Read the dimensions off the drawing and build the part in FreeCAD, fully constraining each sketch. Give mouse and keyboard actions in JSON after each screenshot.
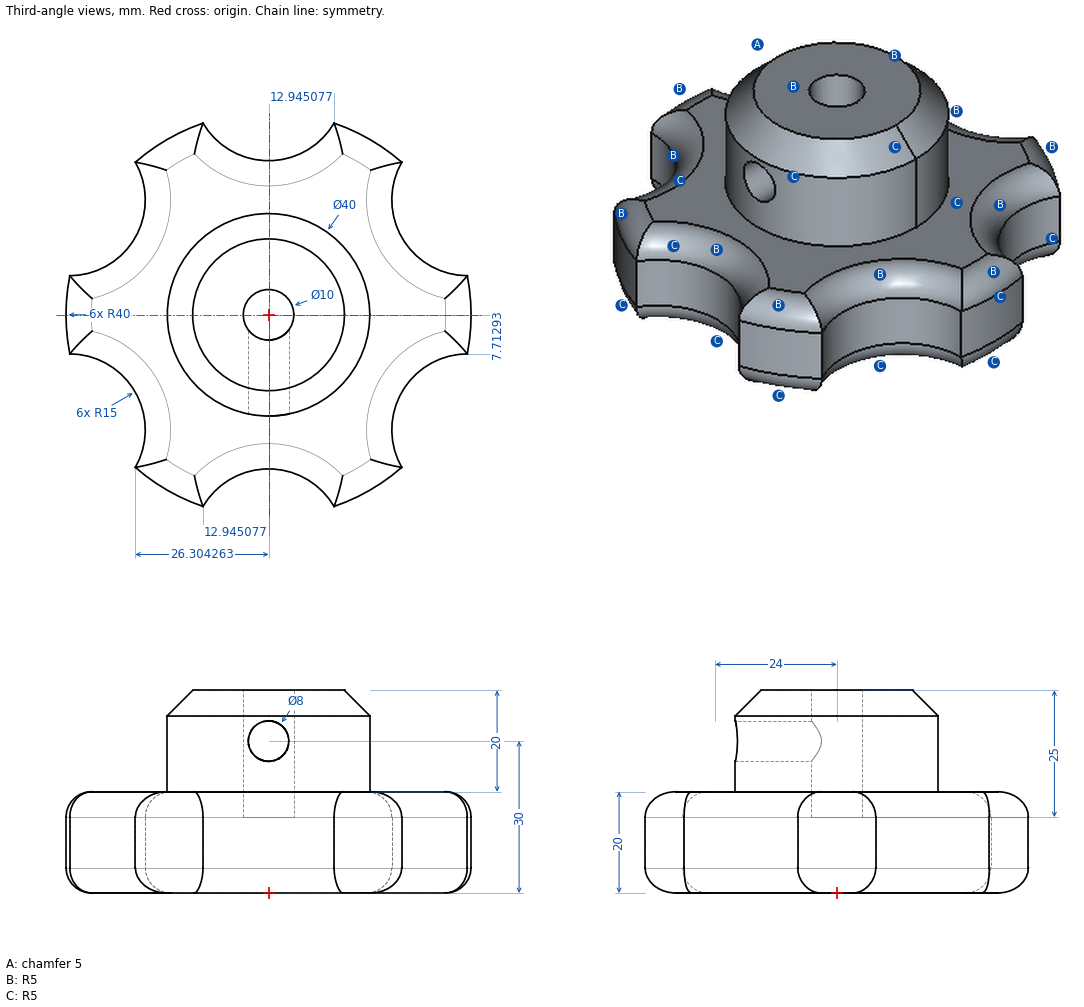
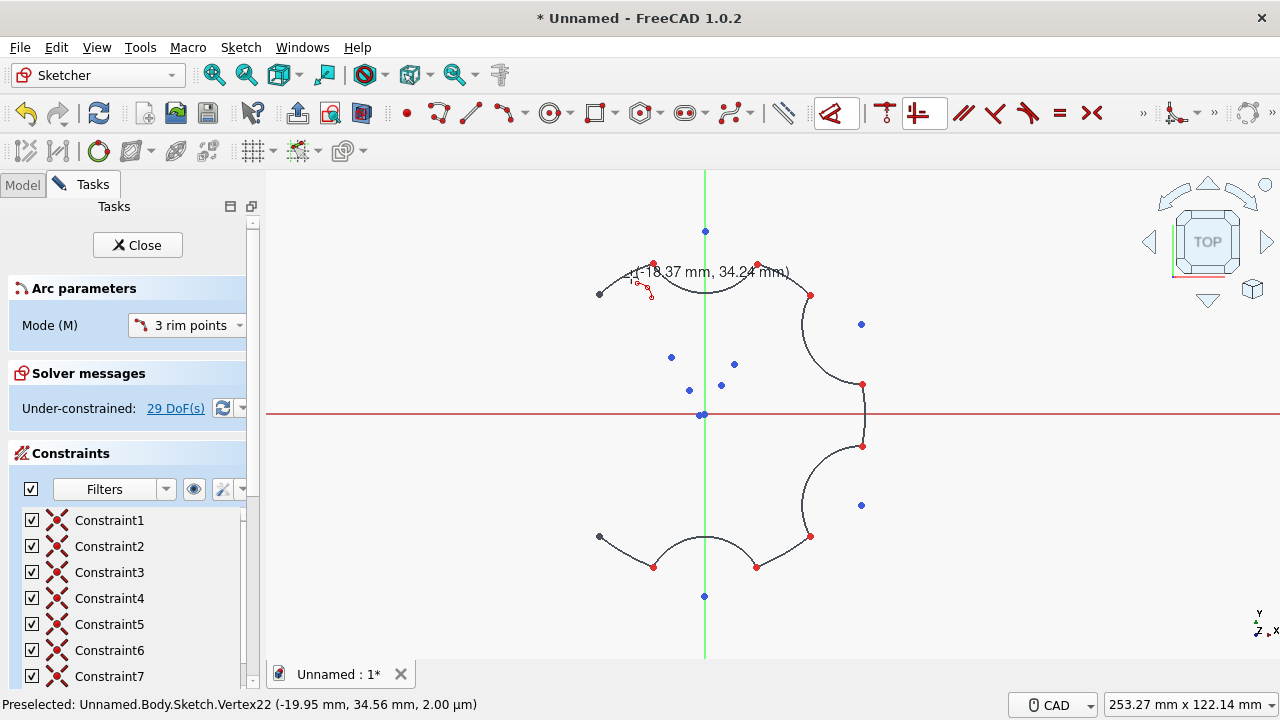
{"action": "left_click", "coordinate": [600, 294]}
{"action": "left_click", "coordinate": [548, 384]}
{"action": "left_click", "coordinate": [599, 354]}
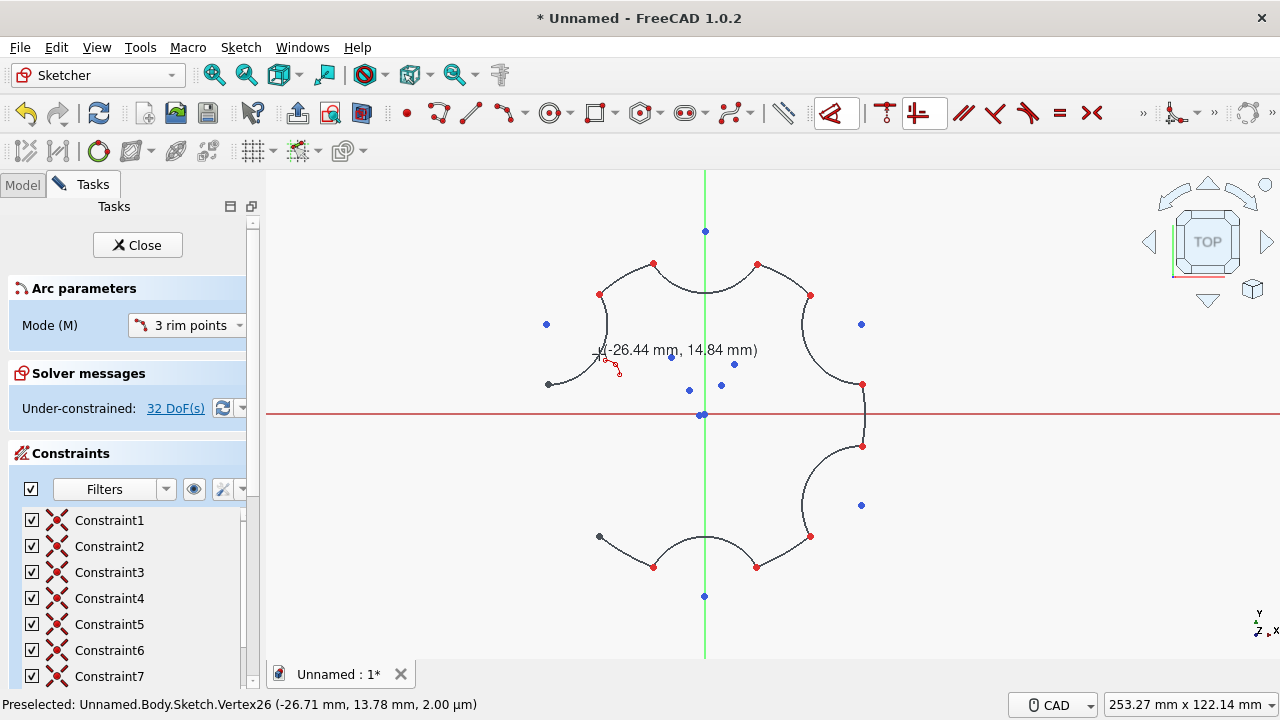
{"action": "left_click", "coordinate": [548, 385]}
{"action": "left_click", "coordinate": [548, 445]}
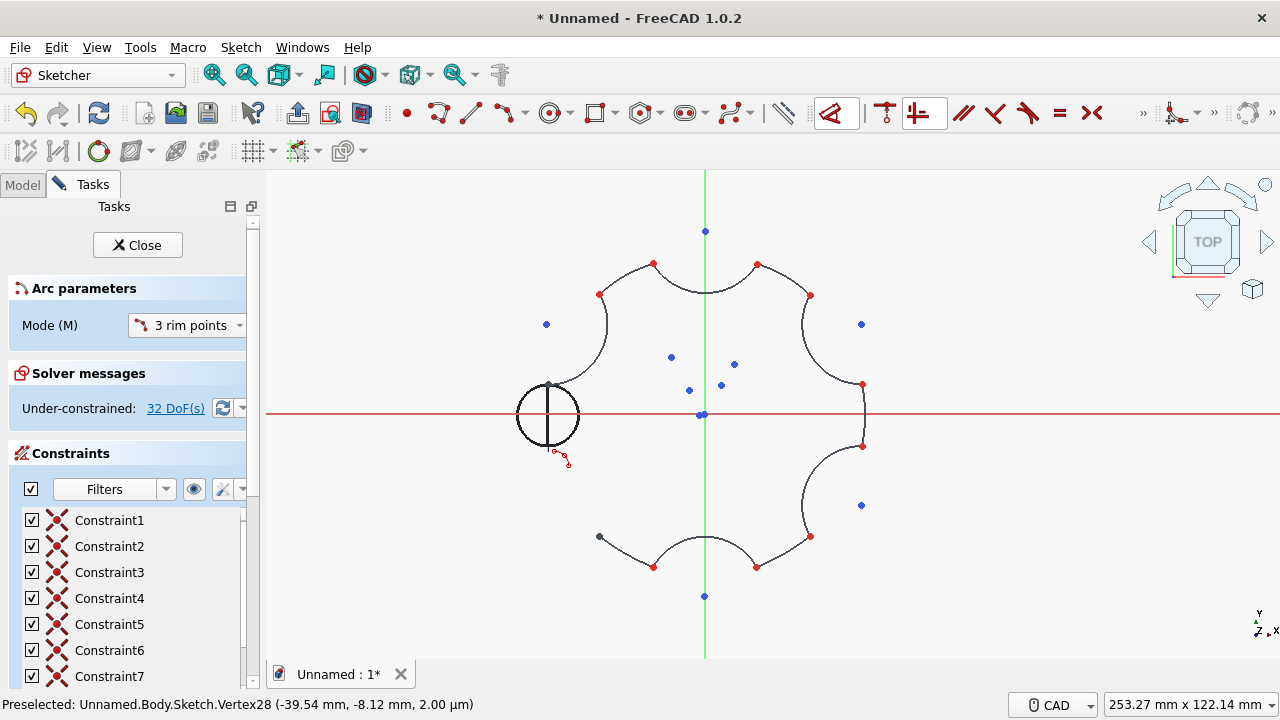
{"action": "scroll", "coordinate": [545, 408], "scroll_direction": "up", "scroll_amount": 9}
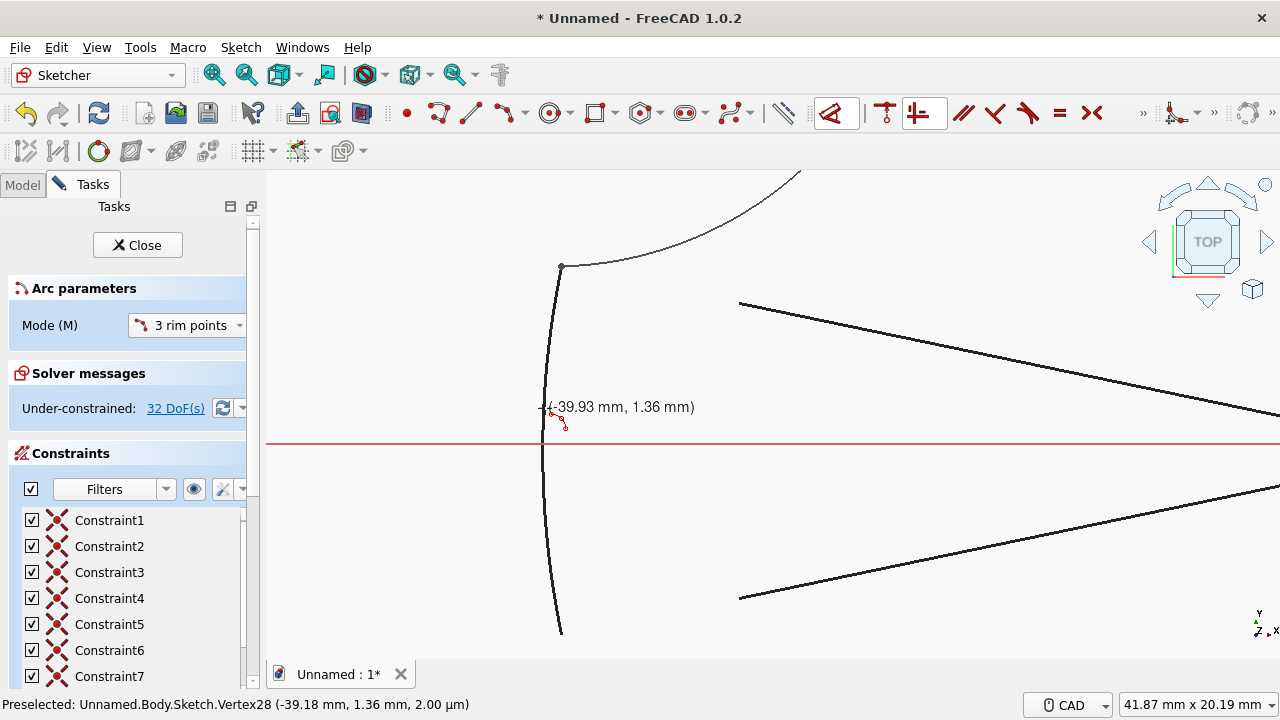
{"action": "left_click", "coordinate": [543, 407]}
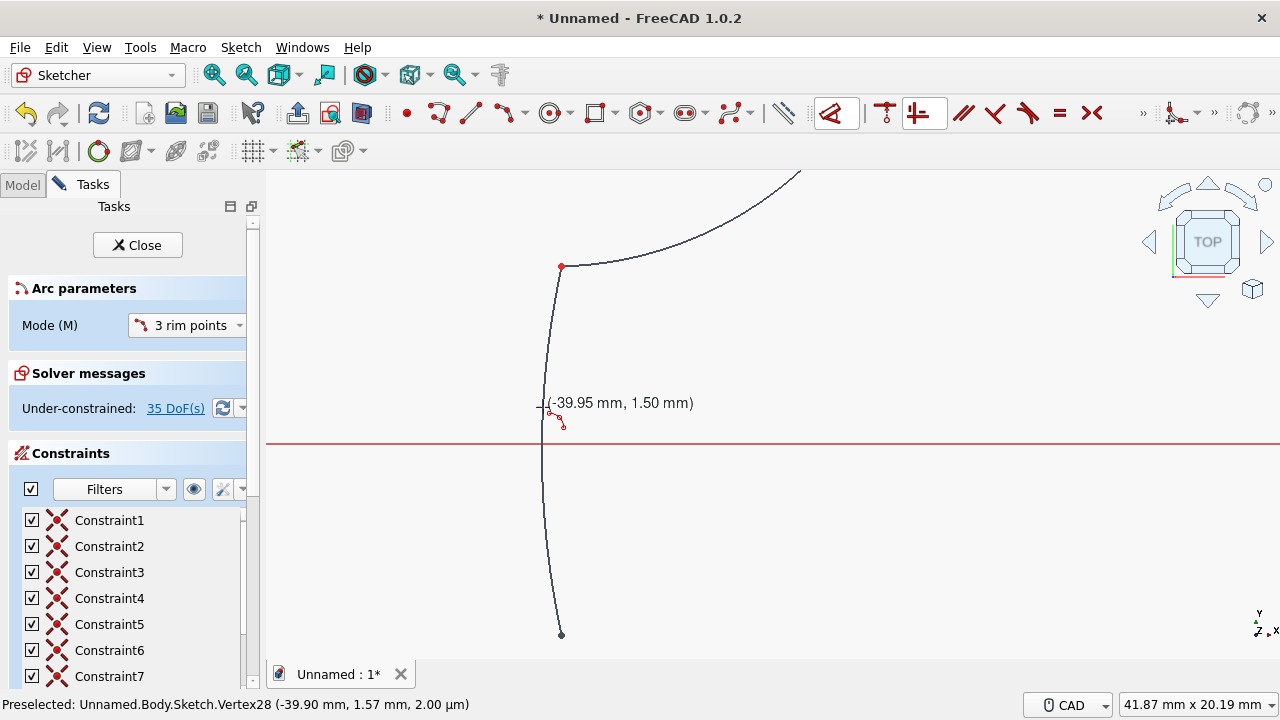
{"action": "scroll", "coordinate": [545, 409], "scroll_direction": "down", "scroll_amount": 9}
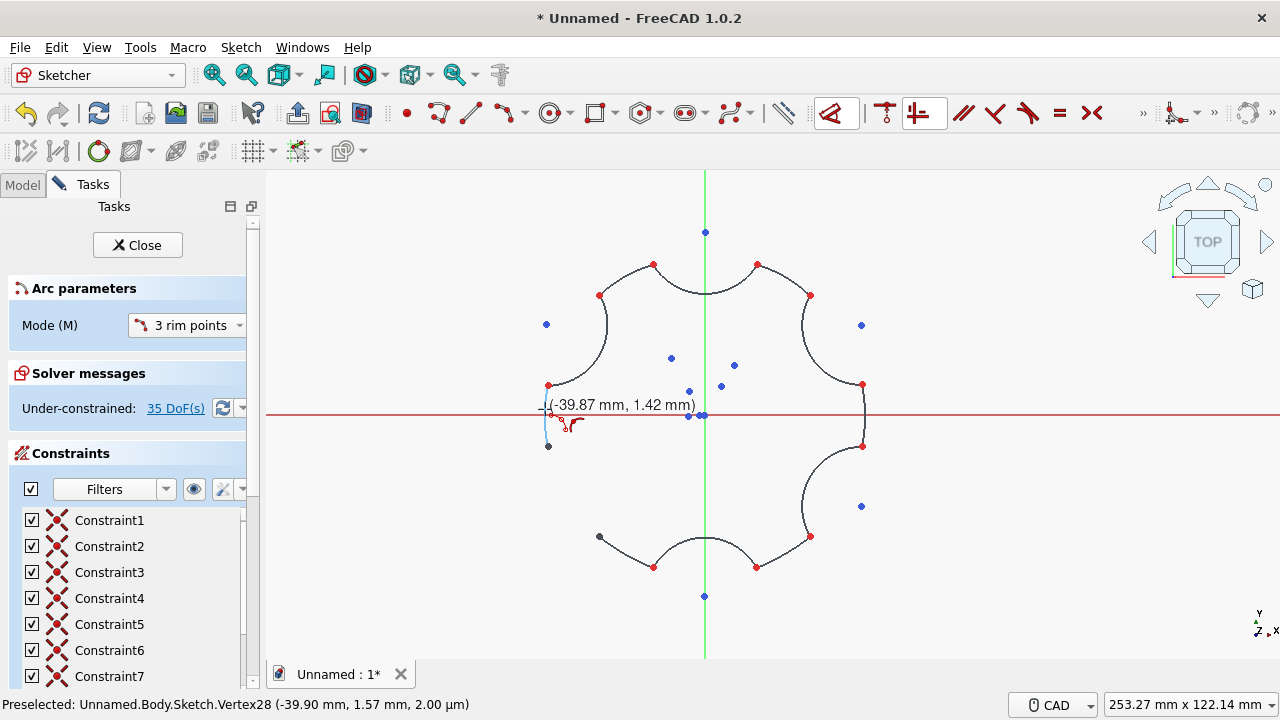
{"action": "left_click", "coordinate": [548, 447]}
{"action": "left_click", "coordinate": [599, 537]}
{"action": "left_click", "coordinate": [599, 476]}
{"action": "key", "text": "Escape"}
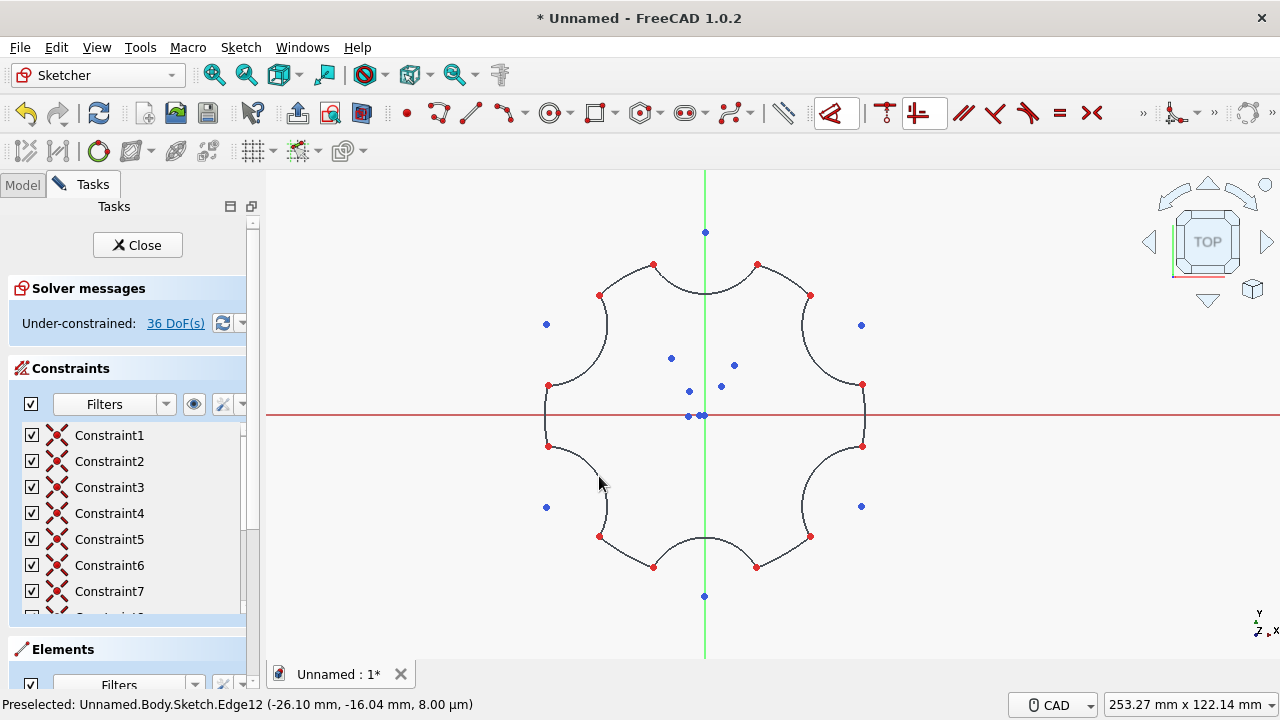
{"action": "left_click", "coordinate": [614, 548]}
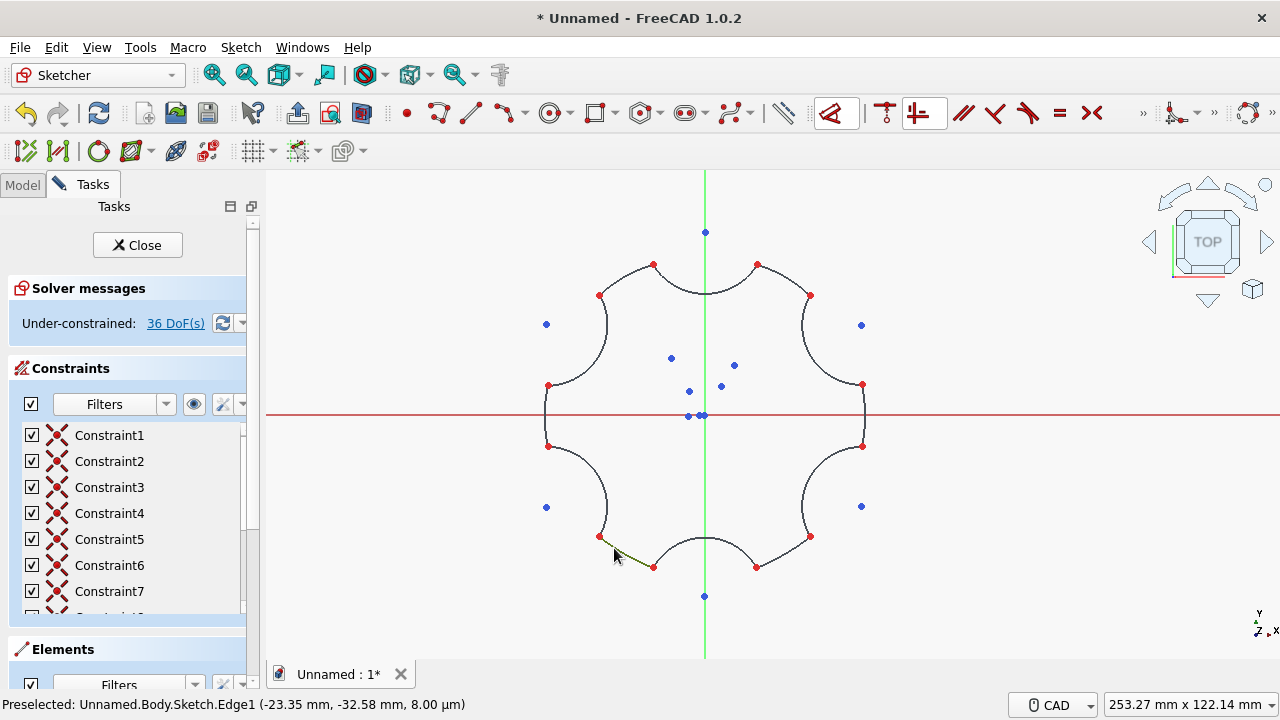
{"action": "left_click", "coordinate": [774, 560]}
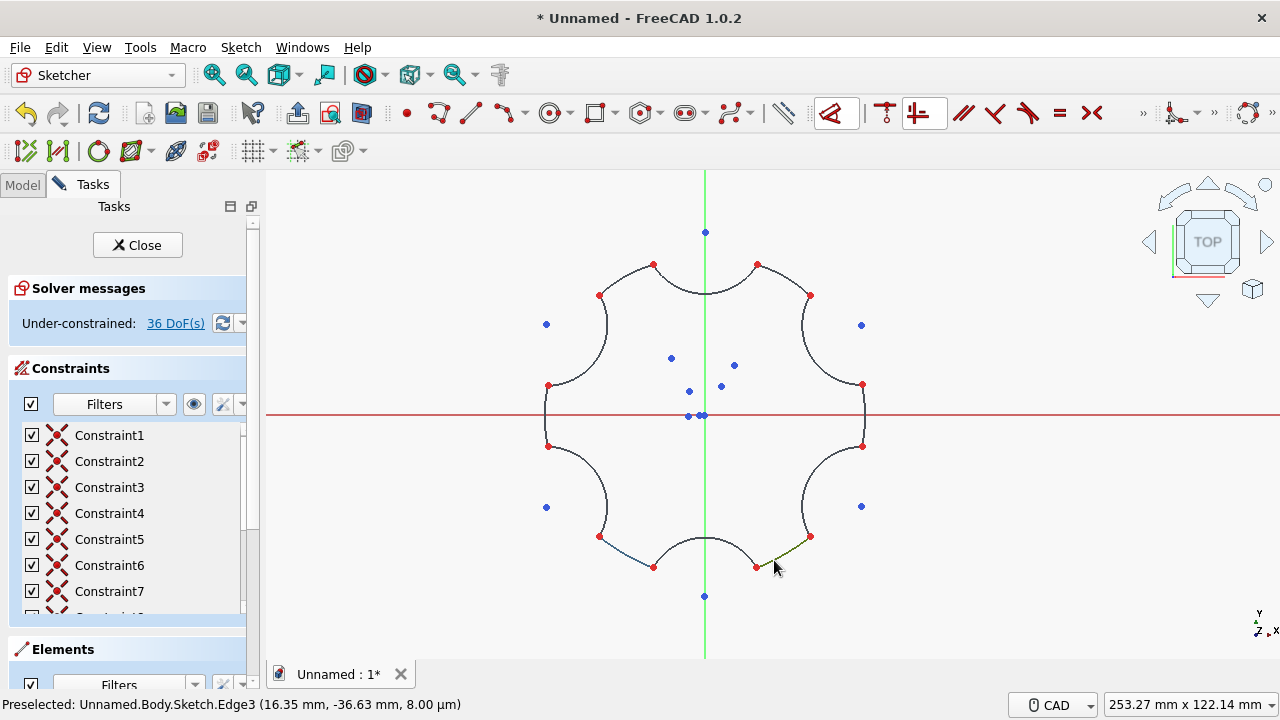
{"action": "left_click", "coordinate": [886, 114]}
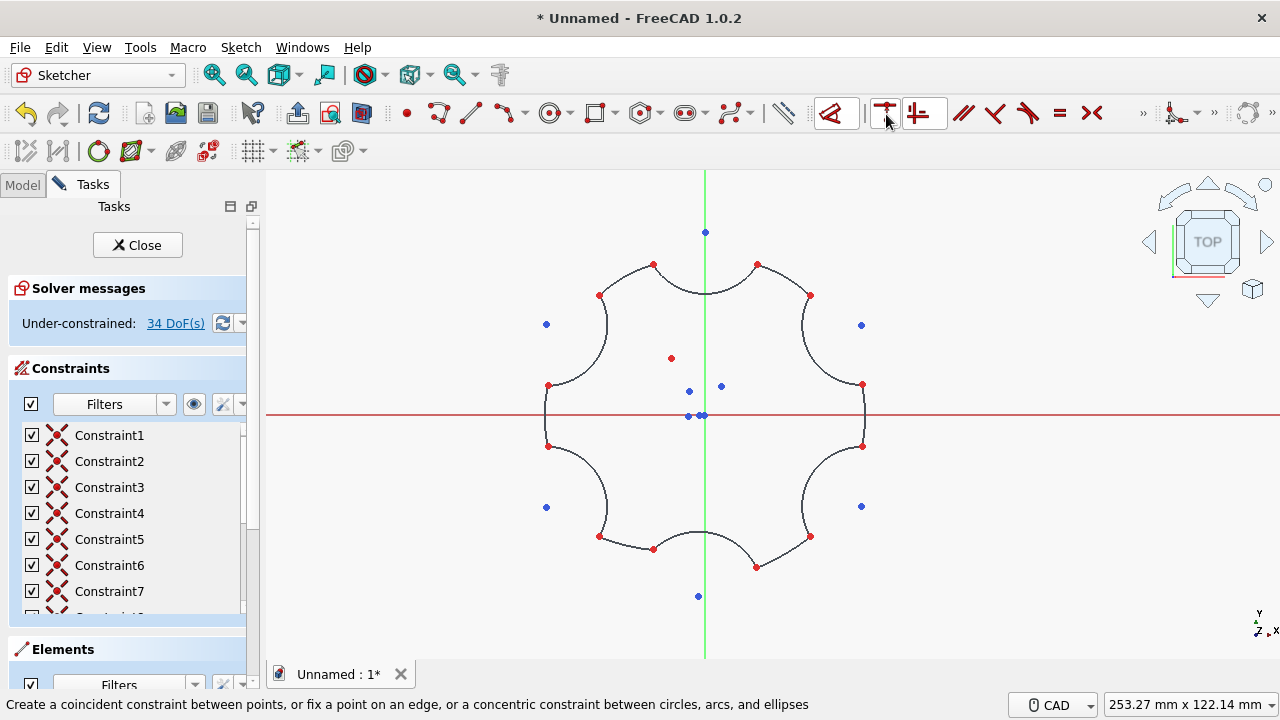
{"action": "left_click", "coordinate": [615, 542]}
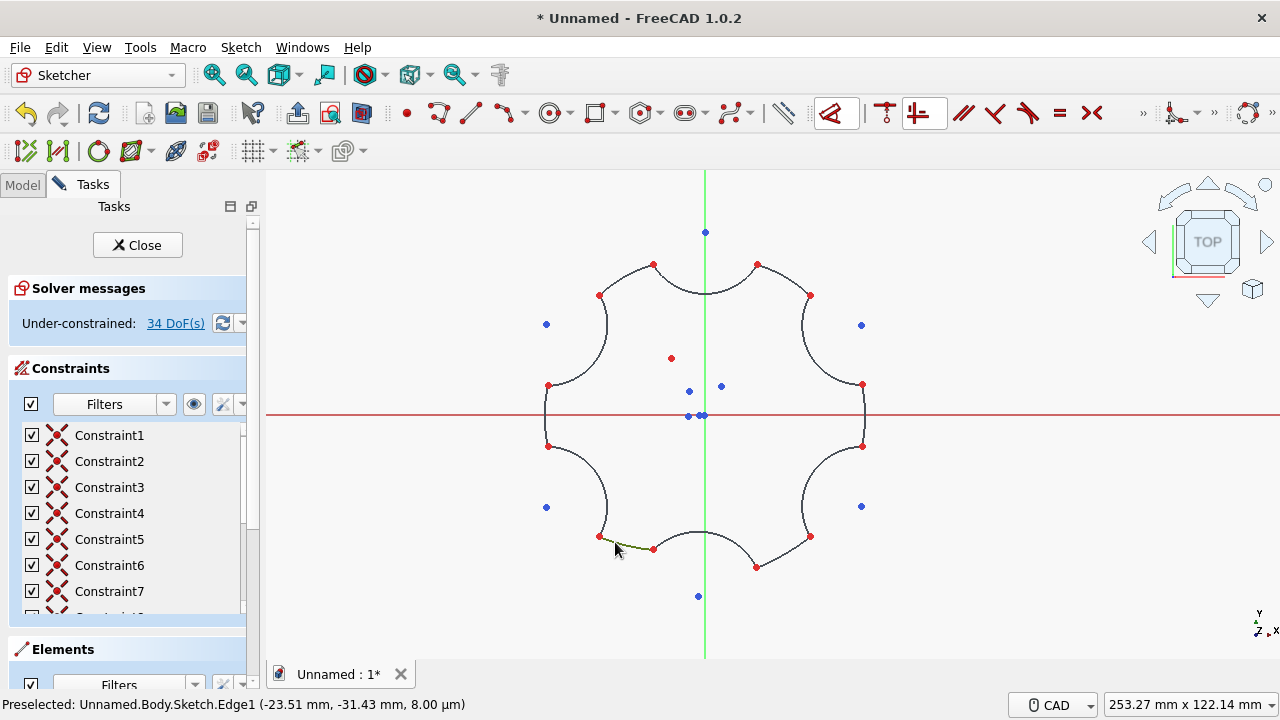
{"action": "left_click", "coordinate": [865, 428]}